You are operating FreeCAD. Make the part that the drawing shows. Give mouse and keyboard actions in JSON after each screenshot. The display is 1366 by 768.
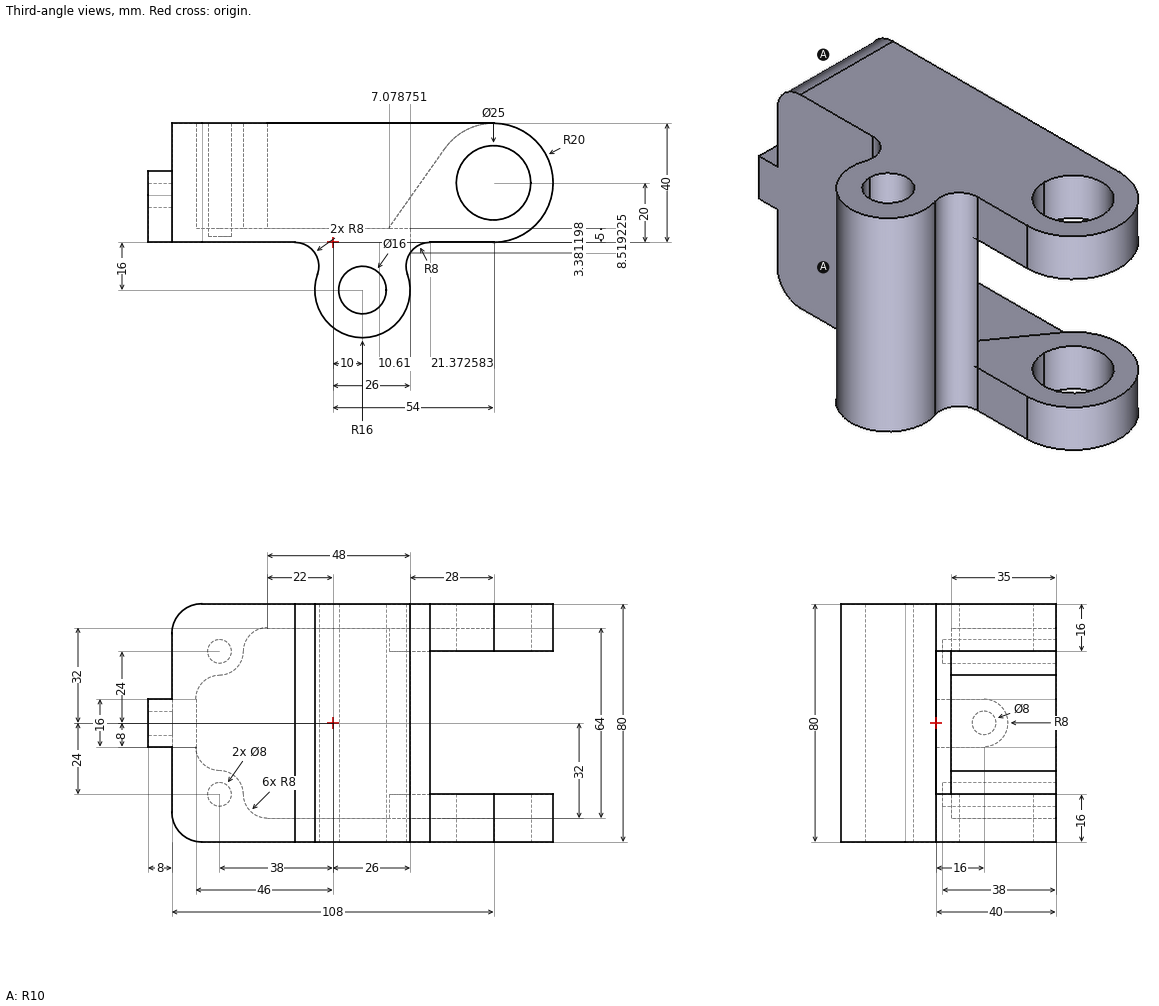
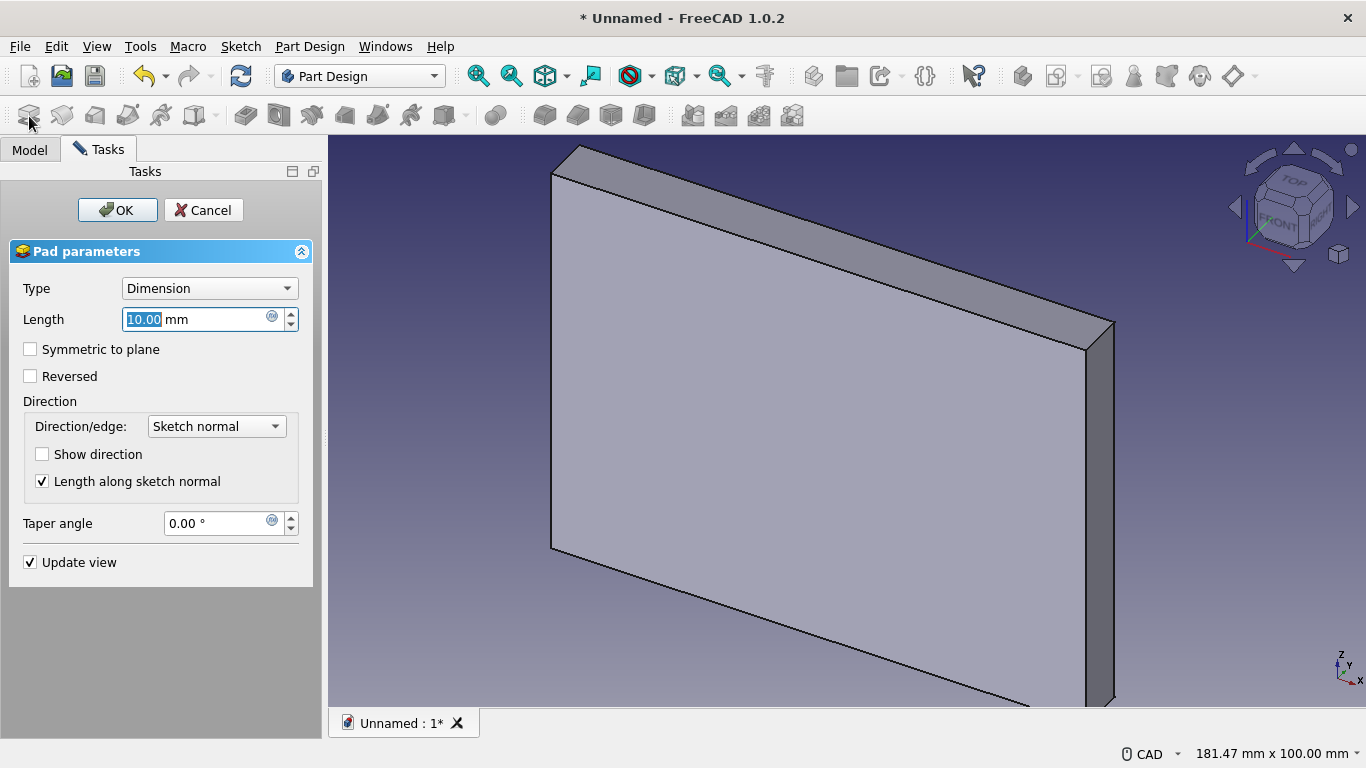
{"action": "type", "text": "40"}
{"action": "key", "text": "Tab"}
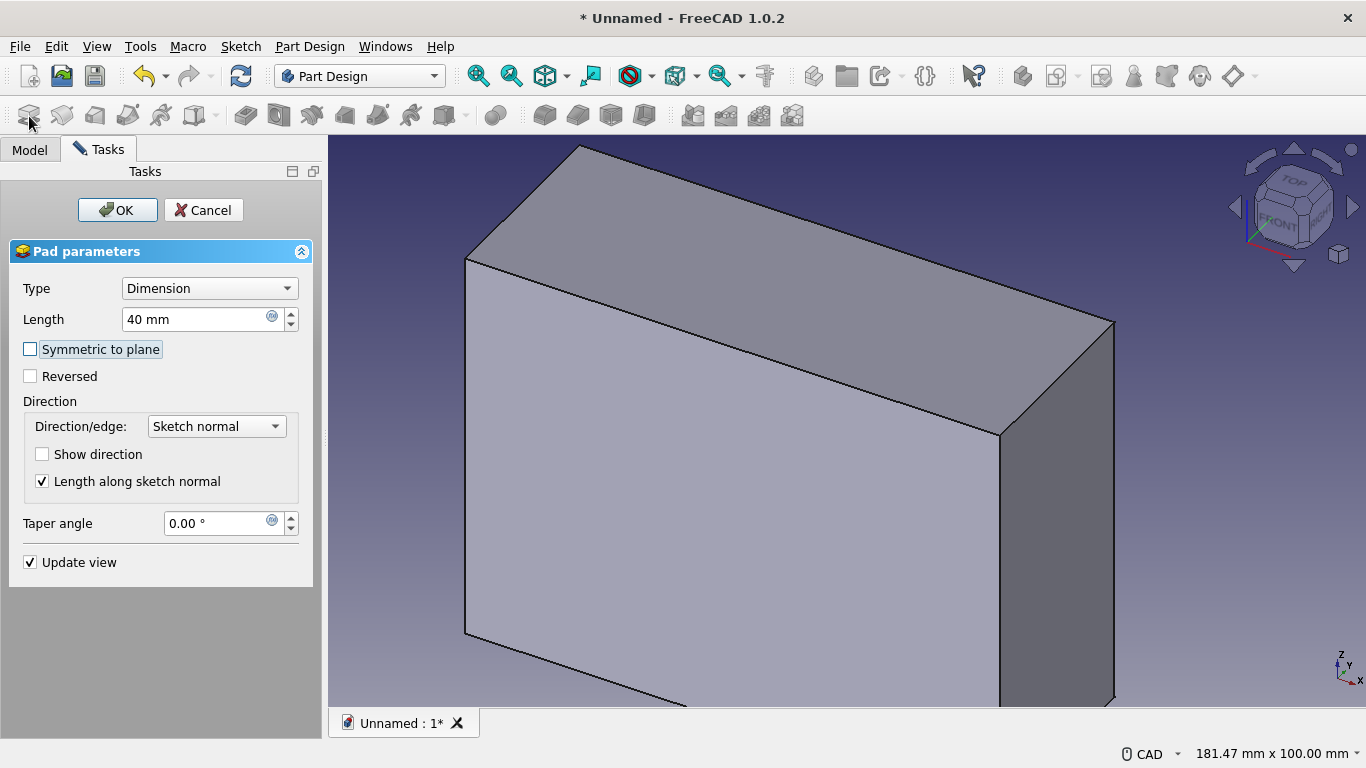
{"action": "left_click", "coordinate": [31, 376]}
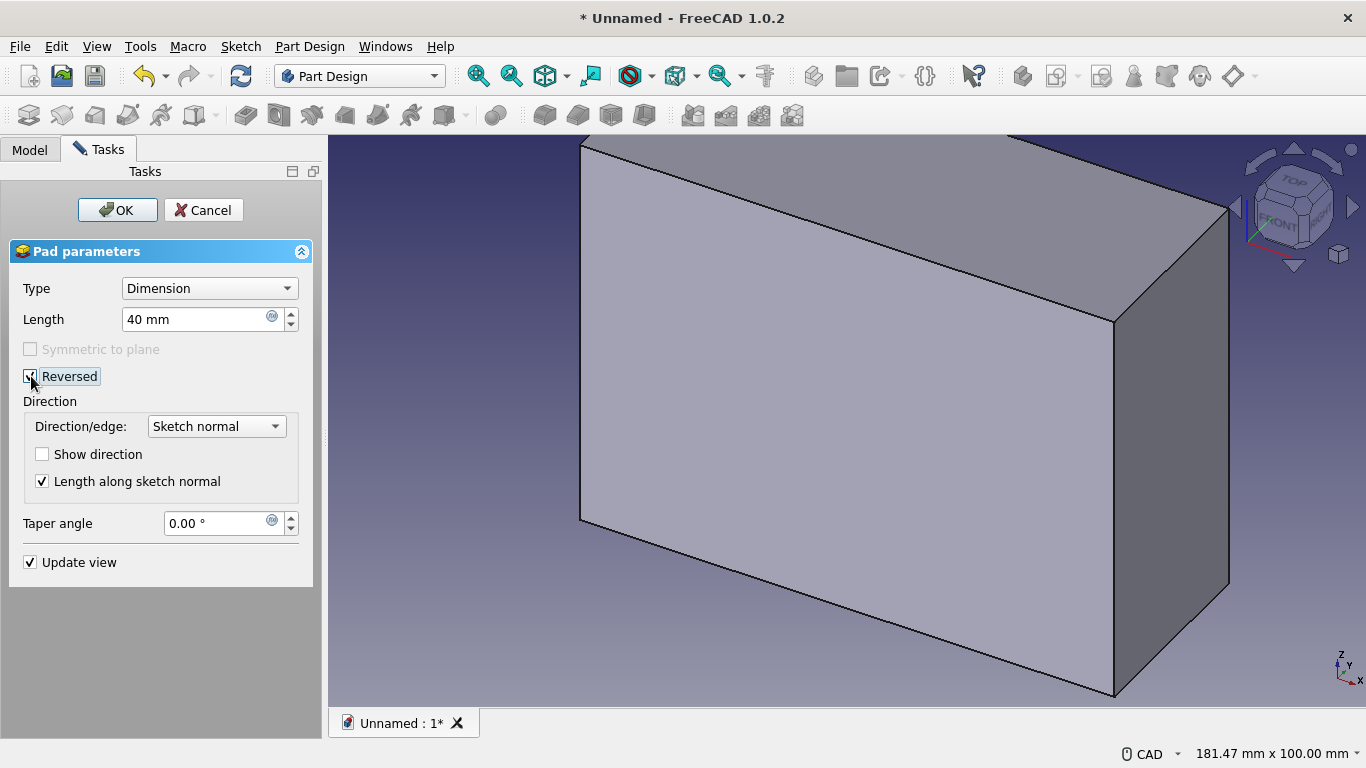
{"action": "left_click", "coordinate": [118, 210]}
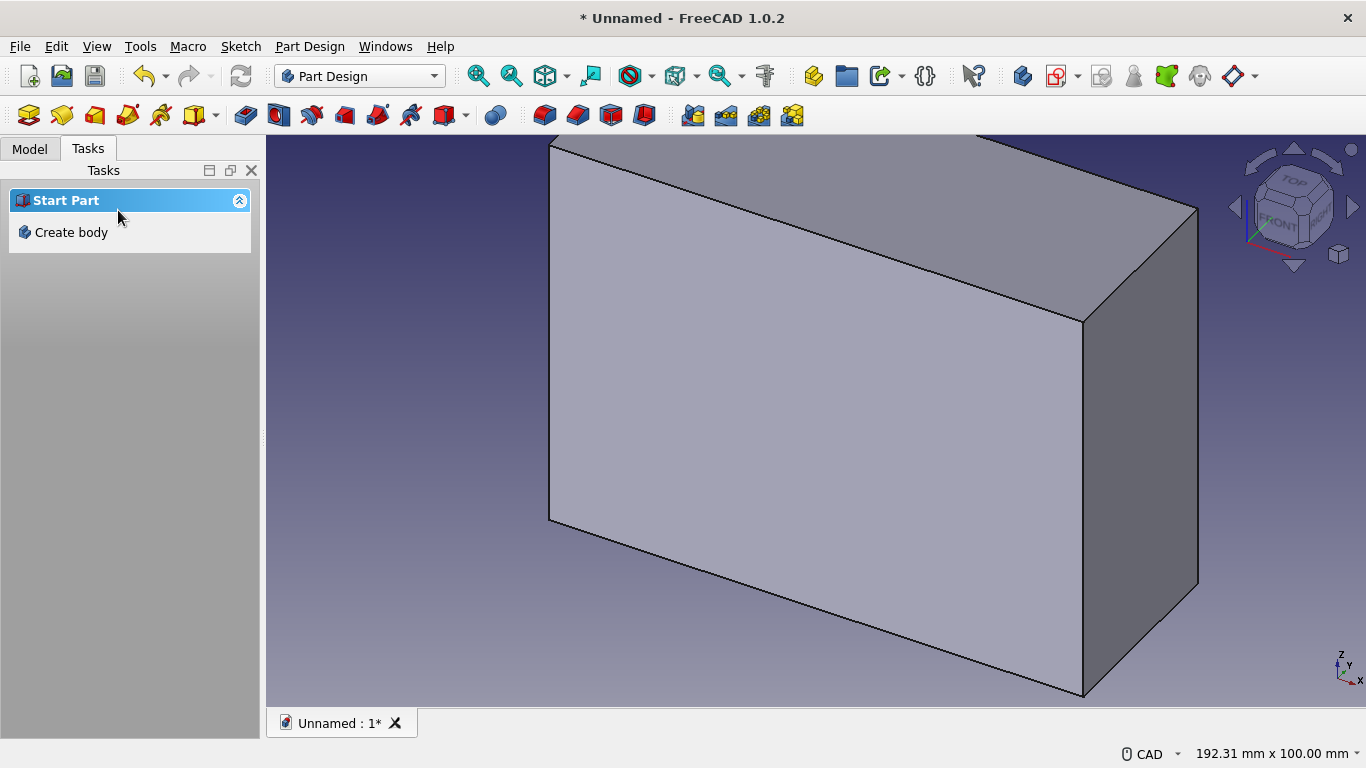
{"action": "key", "text": "v f"}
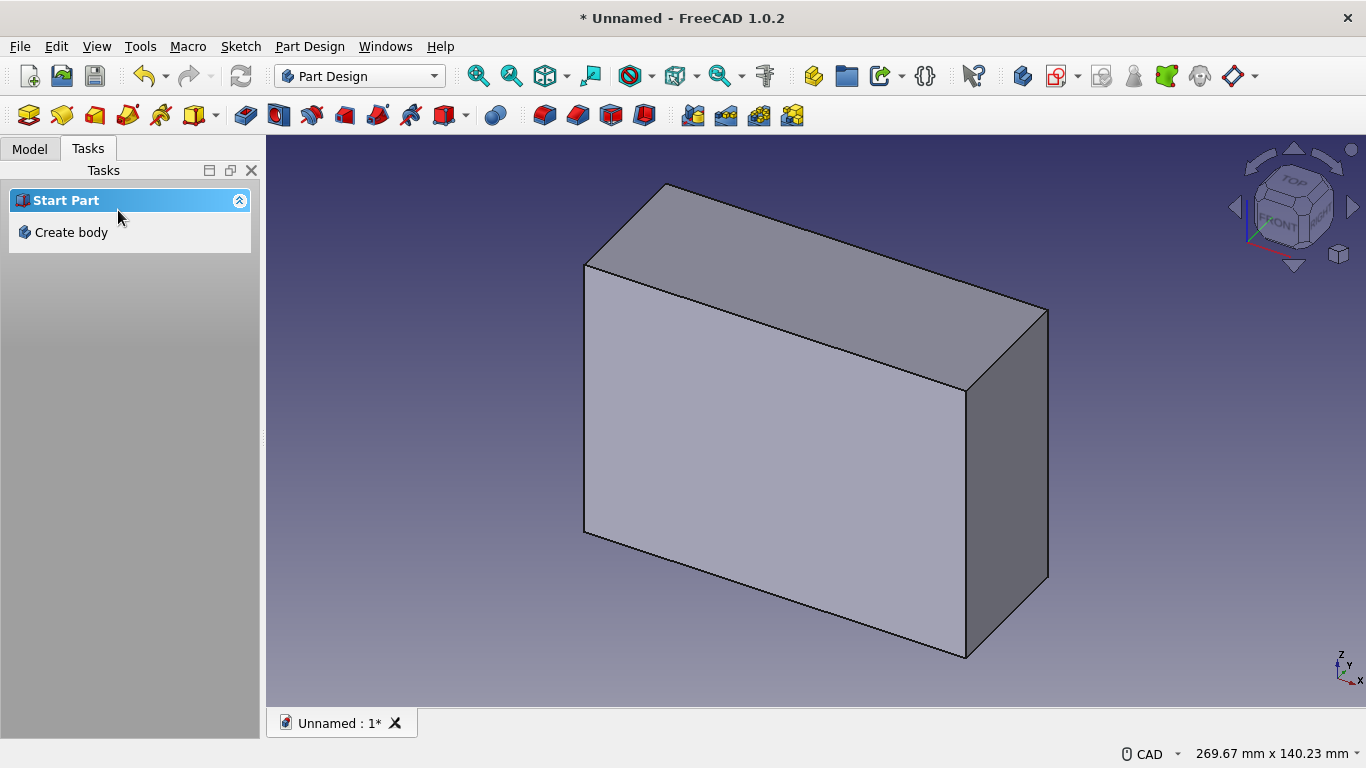
{"action": "key", "text": "4"}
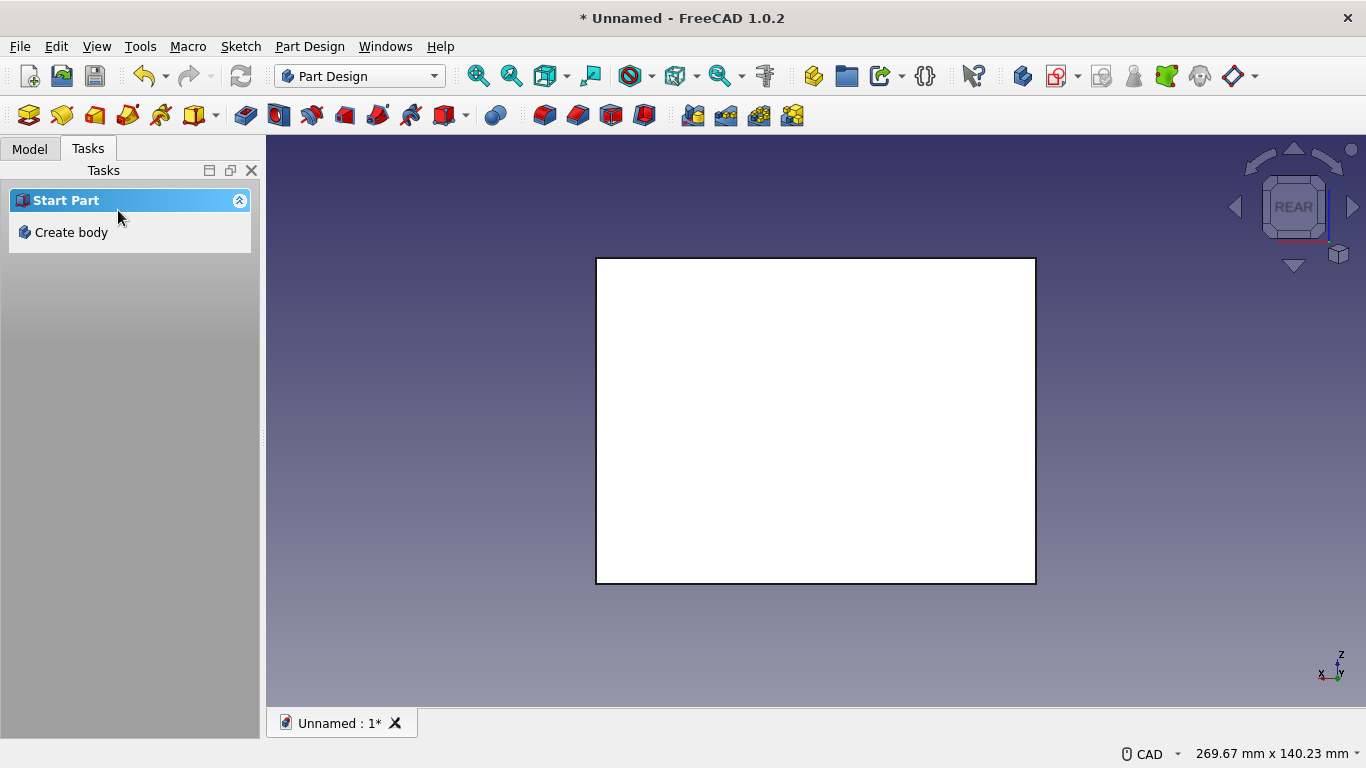
{"action": "left_click", "coordinate": [816, 420]}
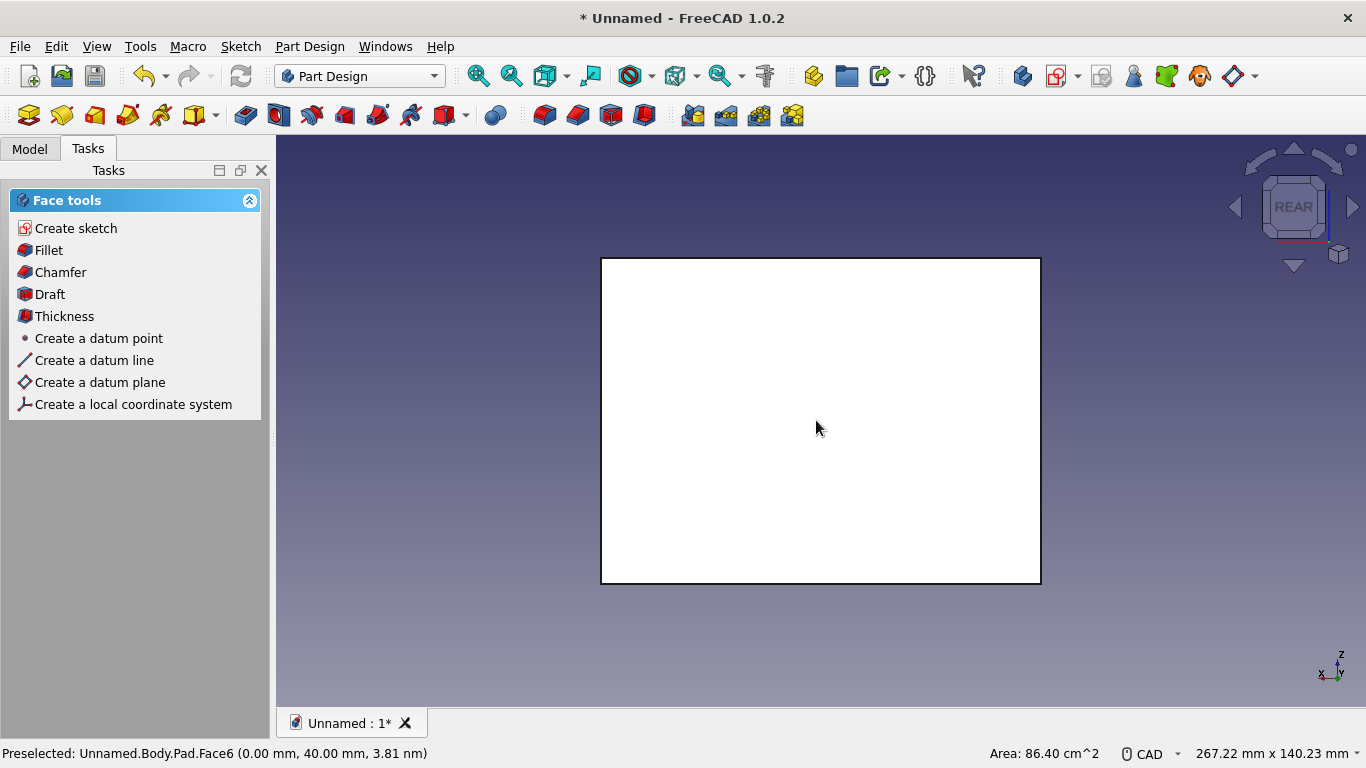
{"action": "left_click", "coordinate": [1056, 76]}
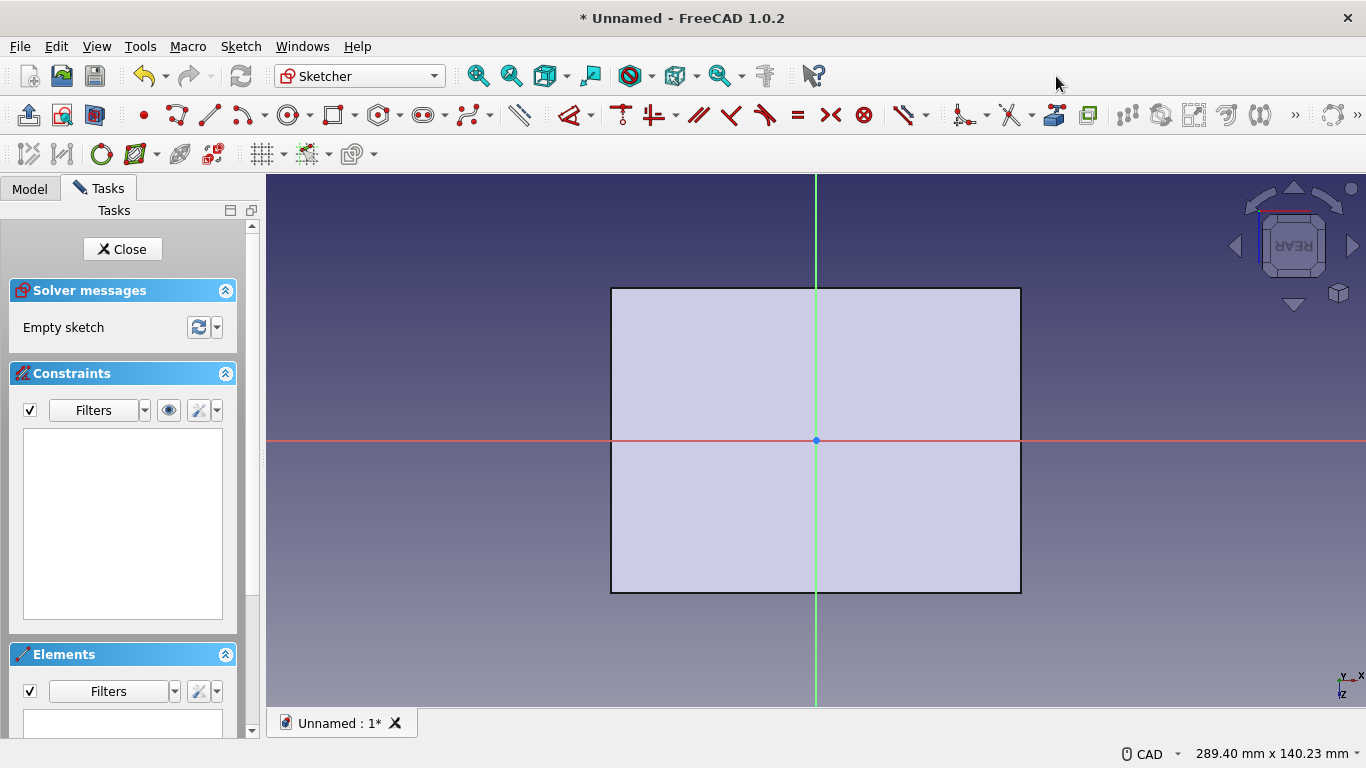
{"action": "scroll", "coordinate": [1201, 441], "scroll_direction": "up", "scroll_amount": 2}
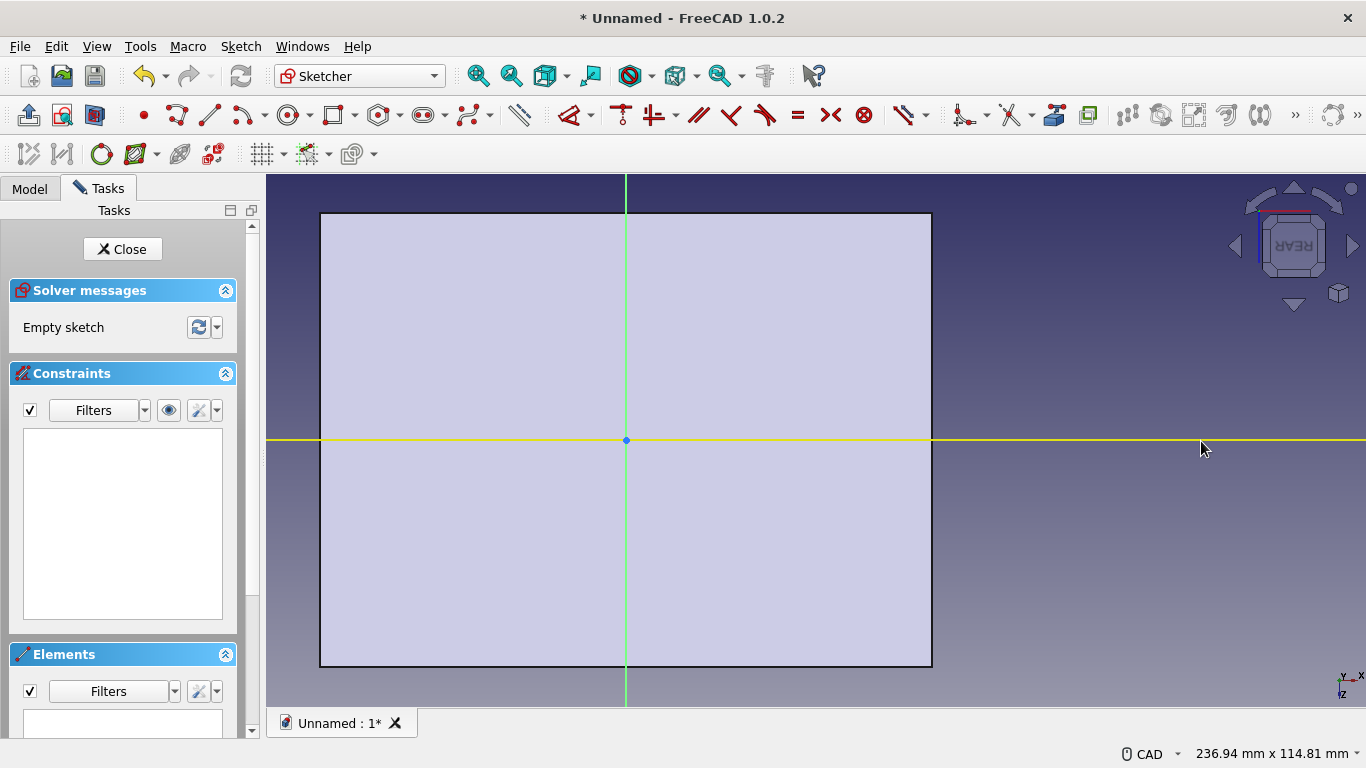
{"action": "key", "text": "g r"}